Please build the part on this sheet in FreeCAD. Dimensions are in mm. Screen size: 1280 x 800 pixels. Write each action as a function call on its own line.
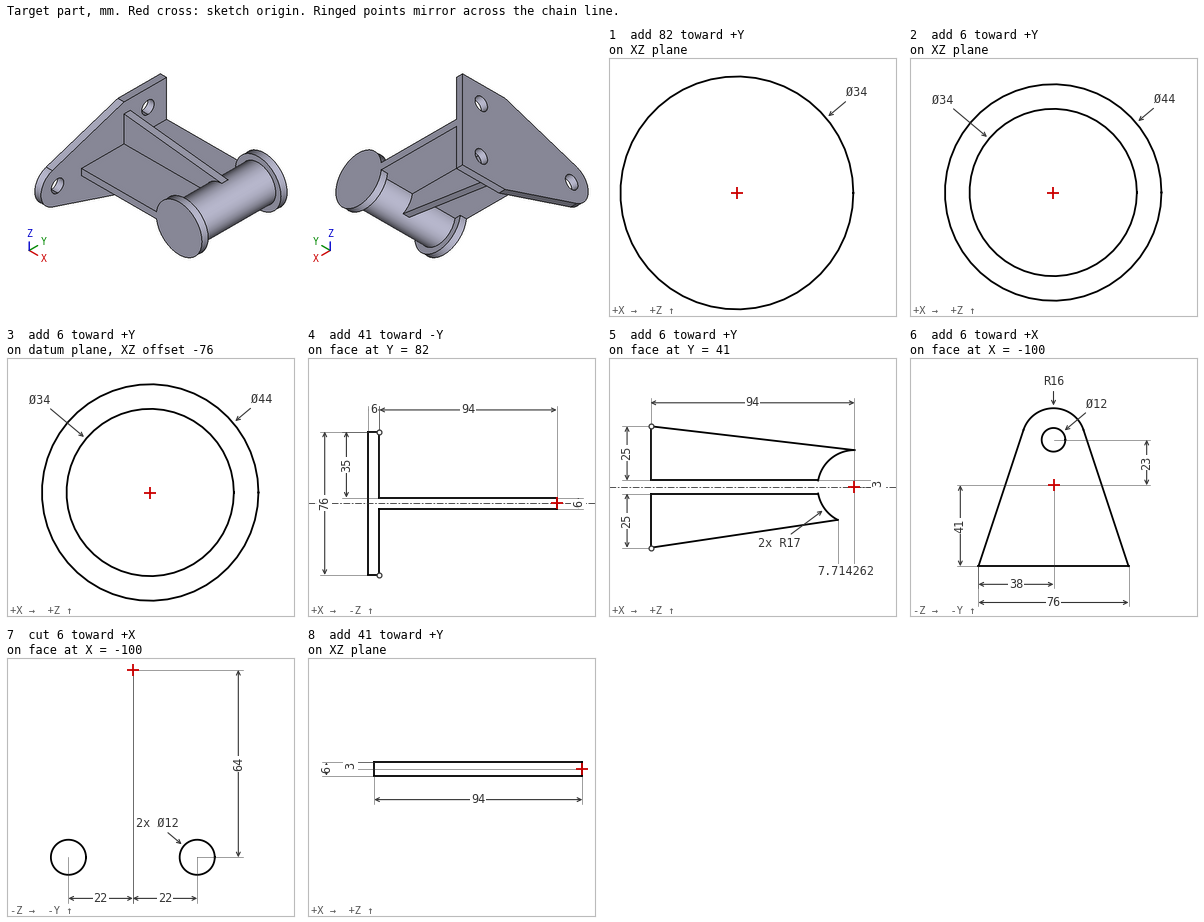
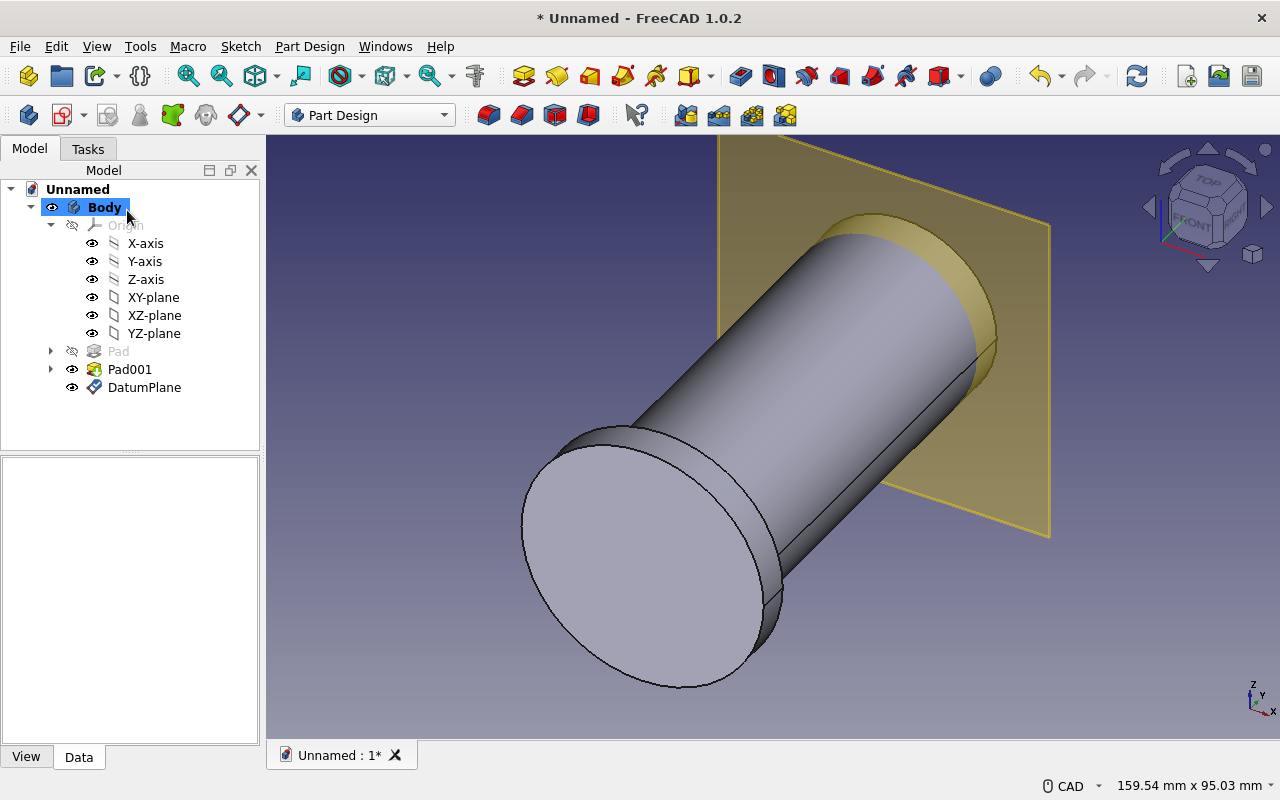
click(117, 387)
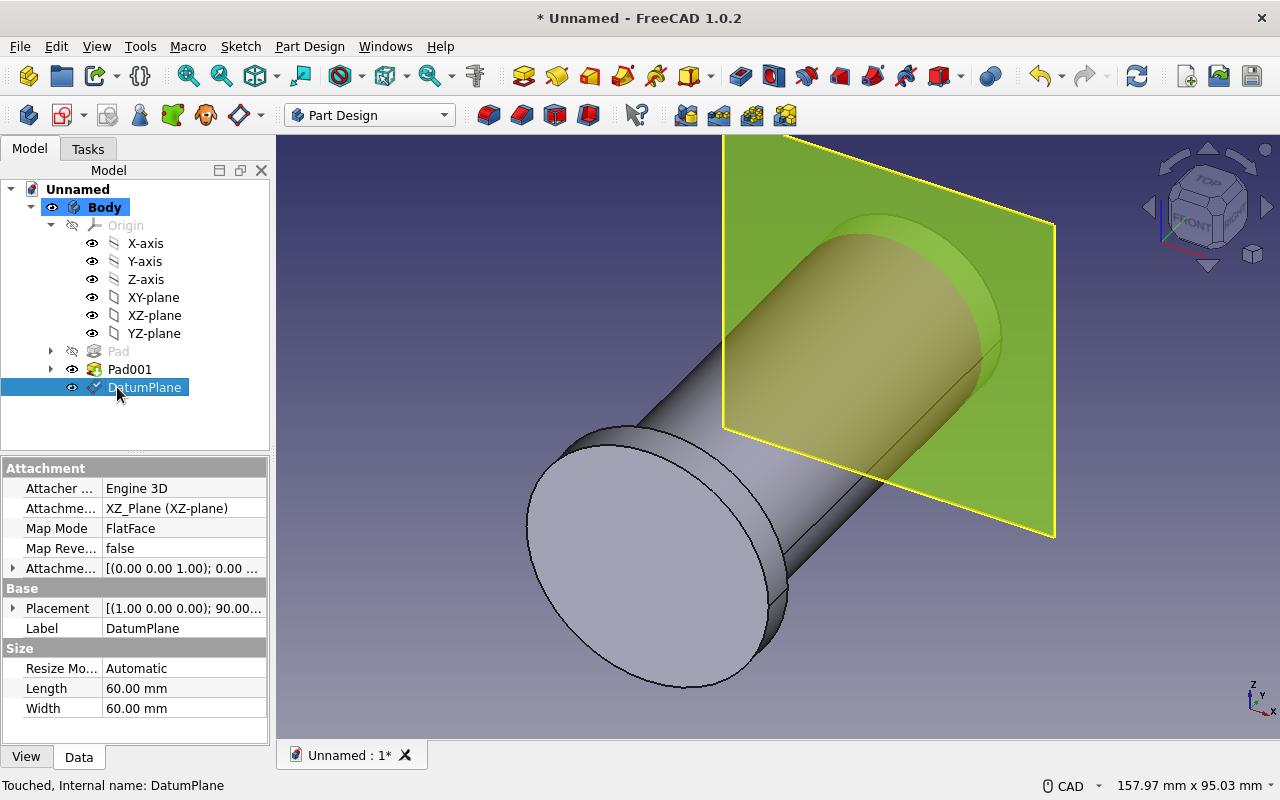
click(62, 116)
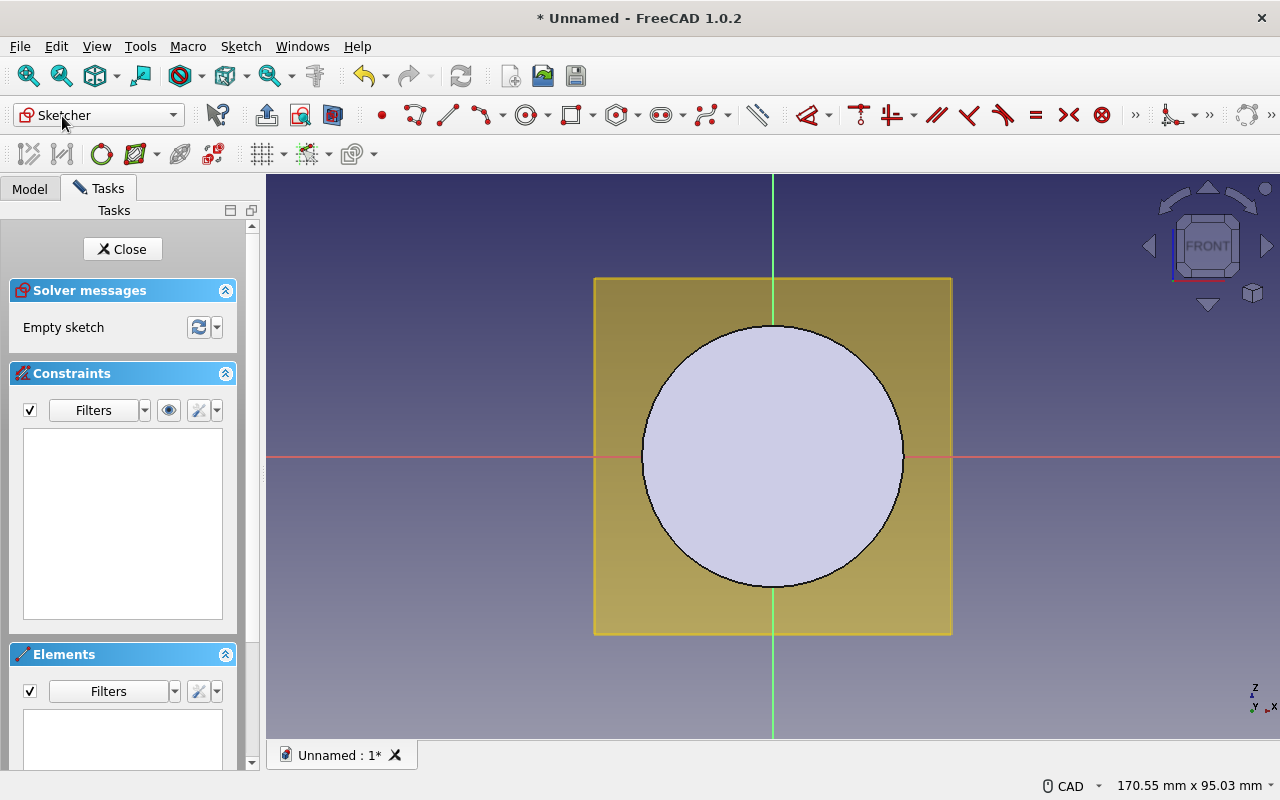
click(333, 116)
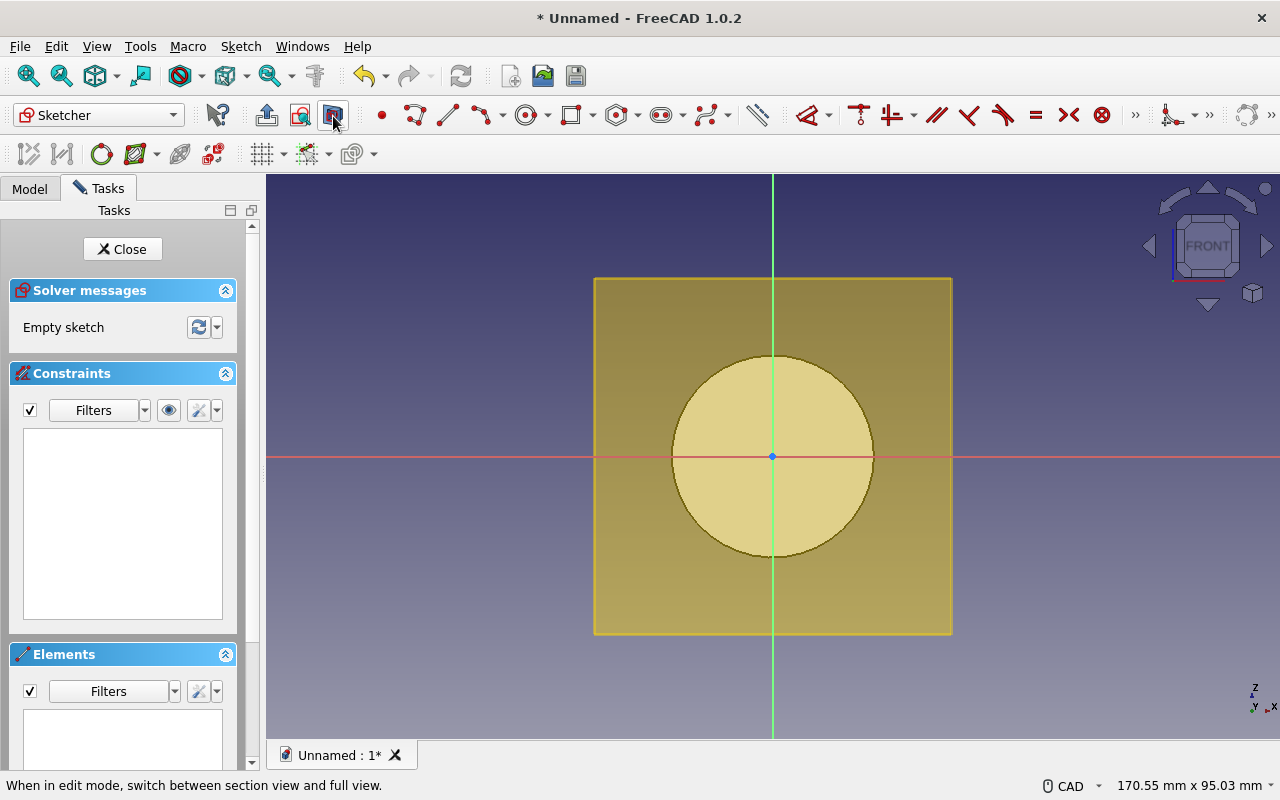
scroll(912, 457, up, 2)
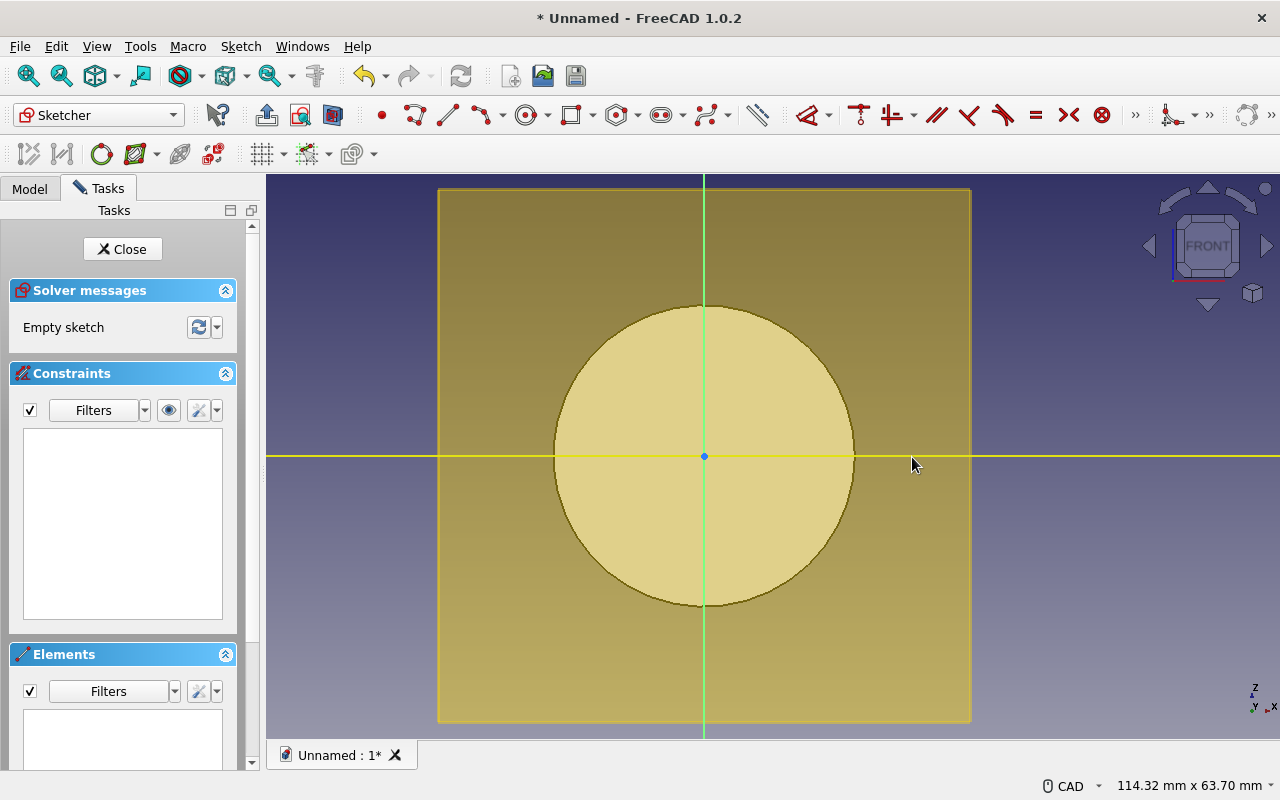
click(526, 116)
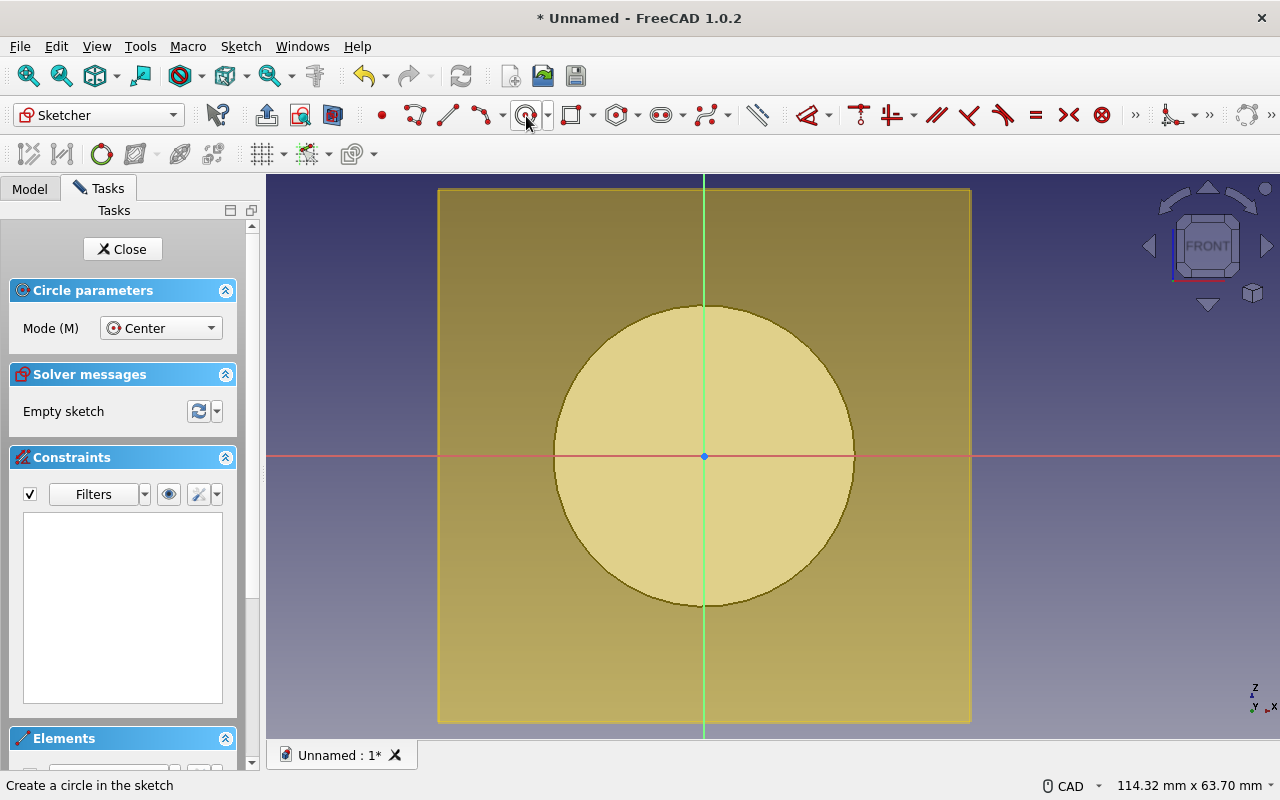
click(704, 456)
click(842, 318)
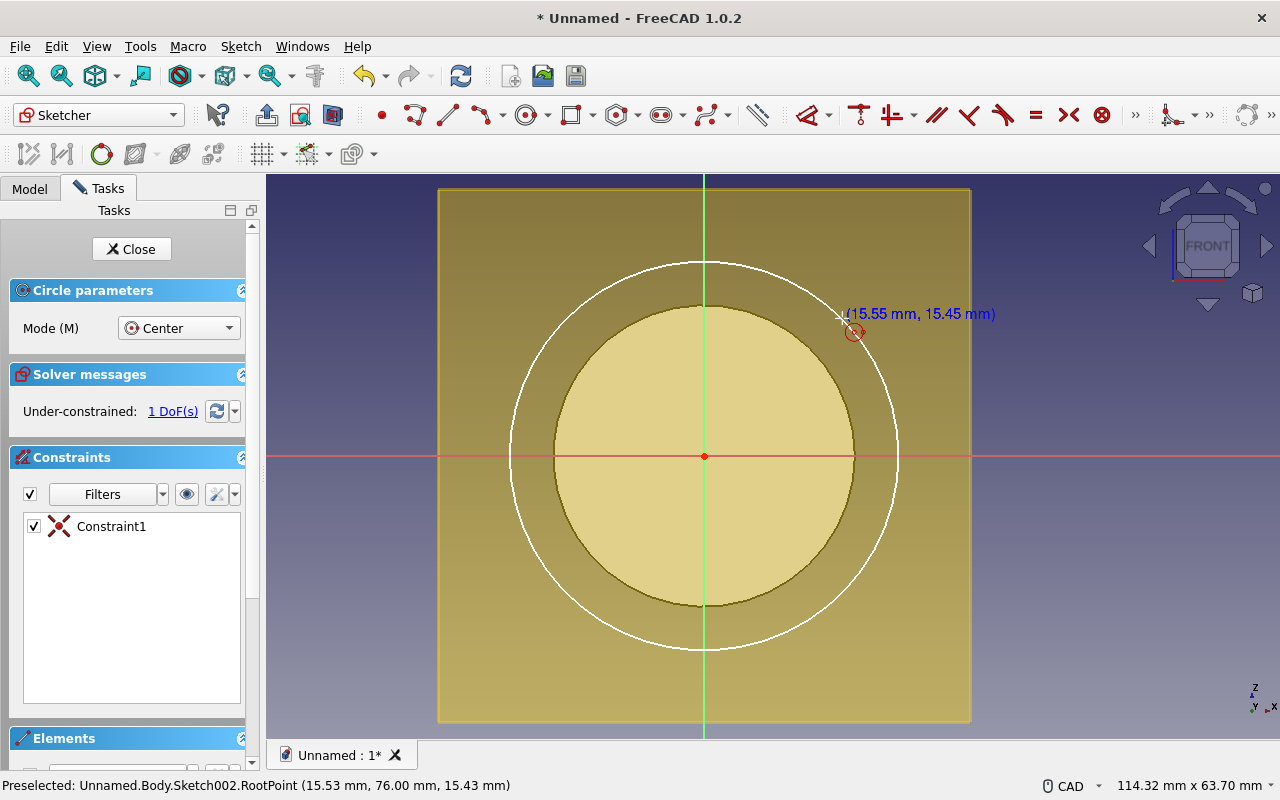
click(704, 456)
click(811, 349)
key(Escape)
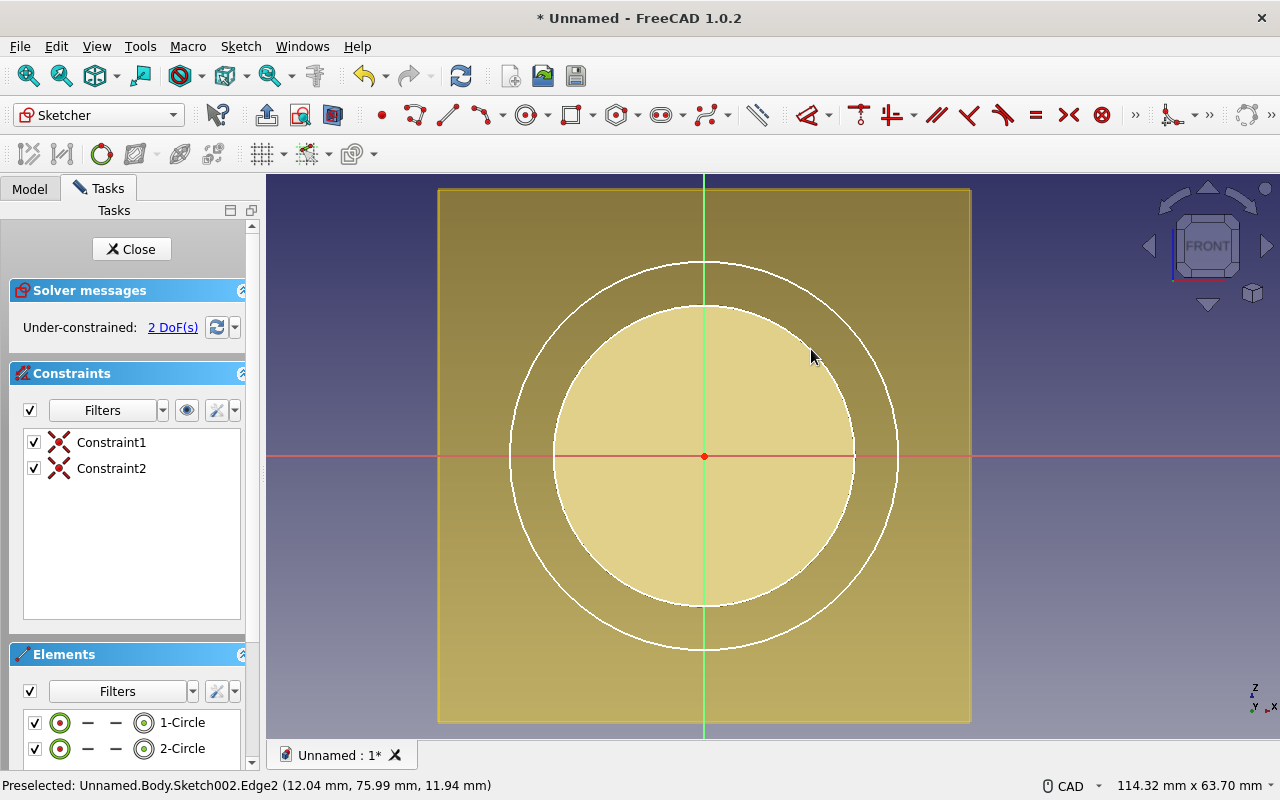
click(806, 116)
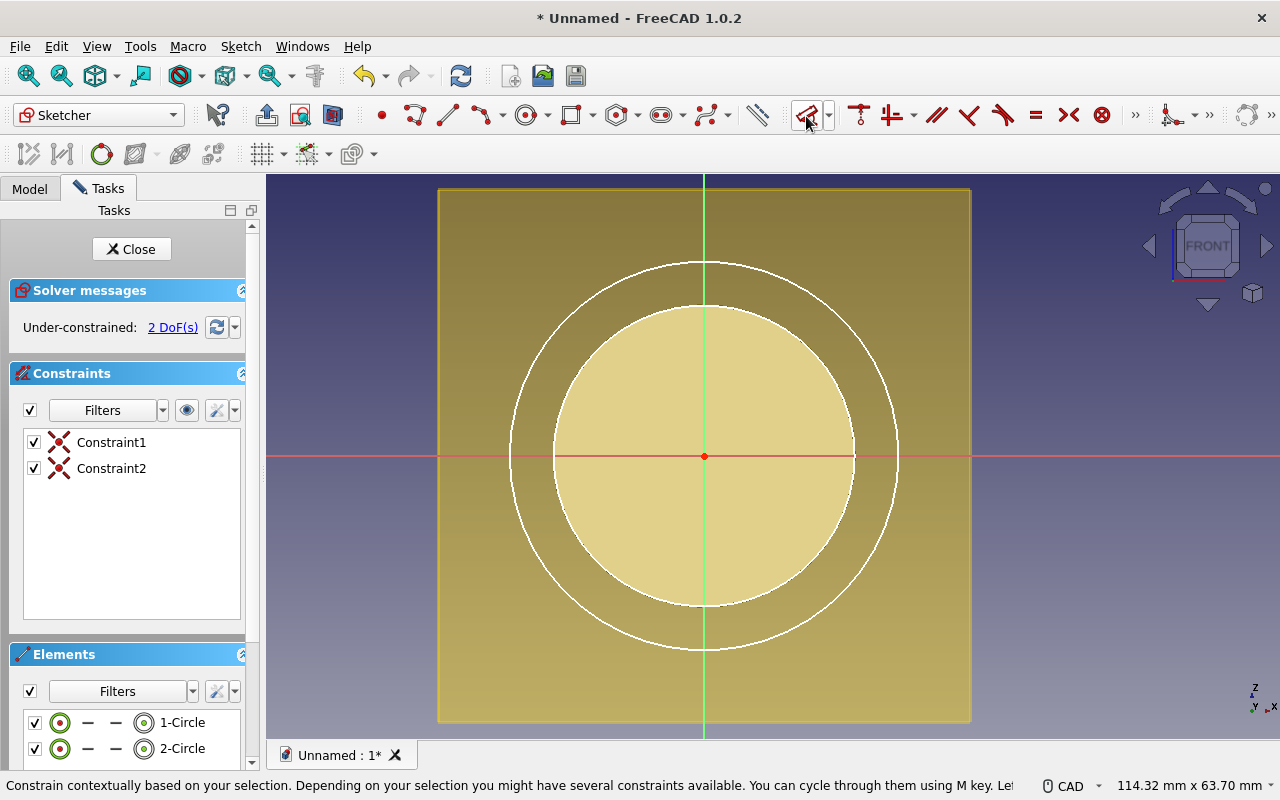
click(841, 318)
click(864, 295)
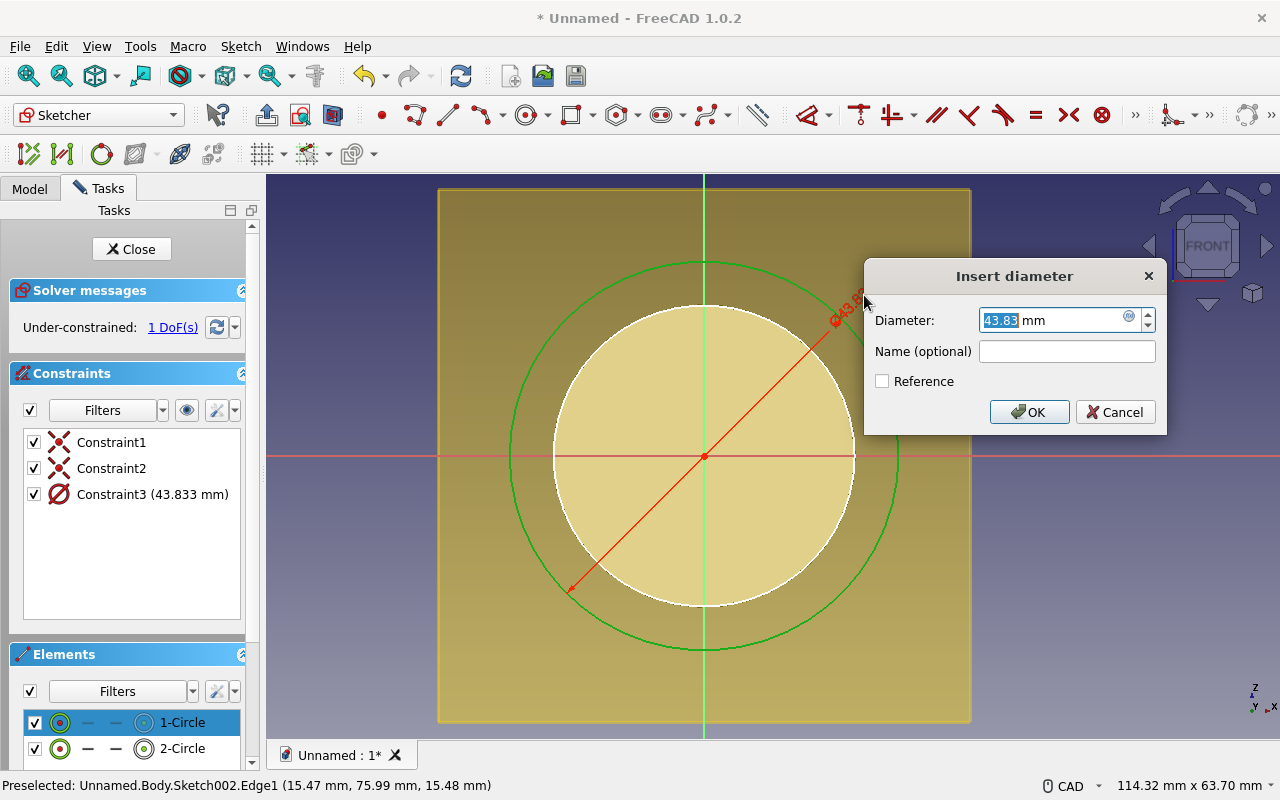
text(44)
key(Return)